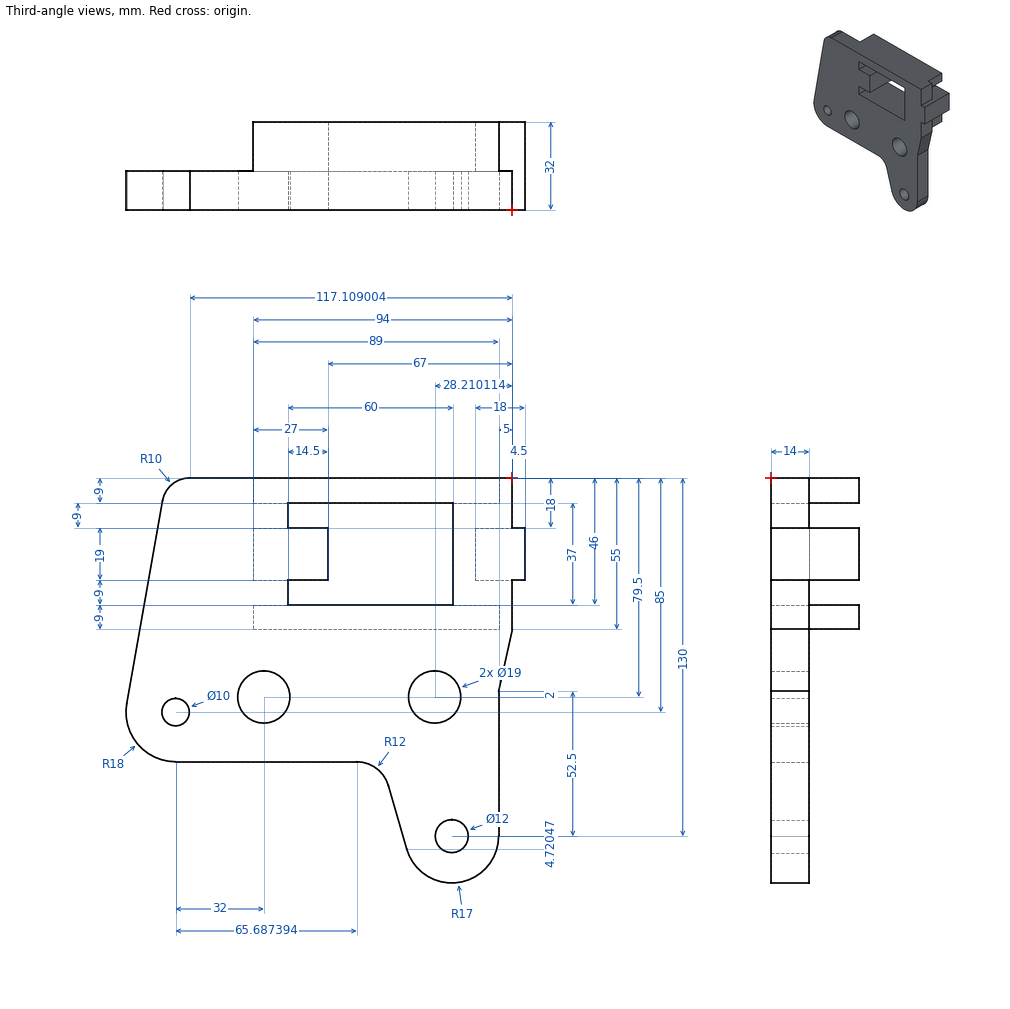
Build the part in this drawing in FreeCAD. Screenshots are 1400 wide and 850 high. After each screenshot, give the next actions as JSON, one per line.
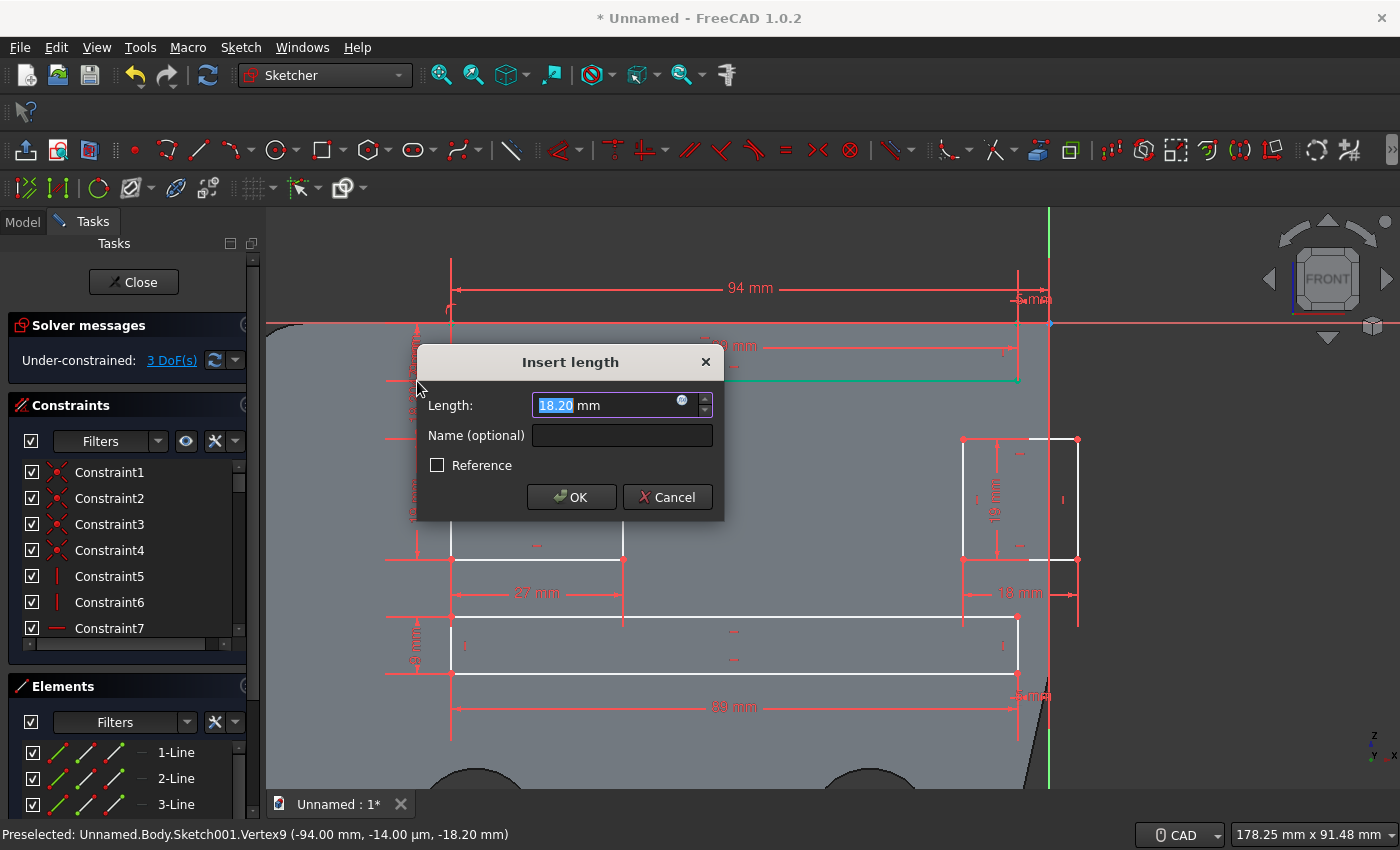
{"action": "type", "text": "18"}
{"action": "key", "text": "Return"}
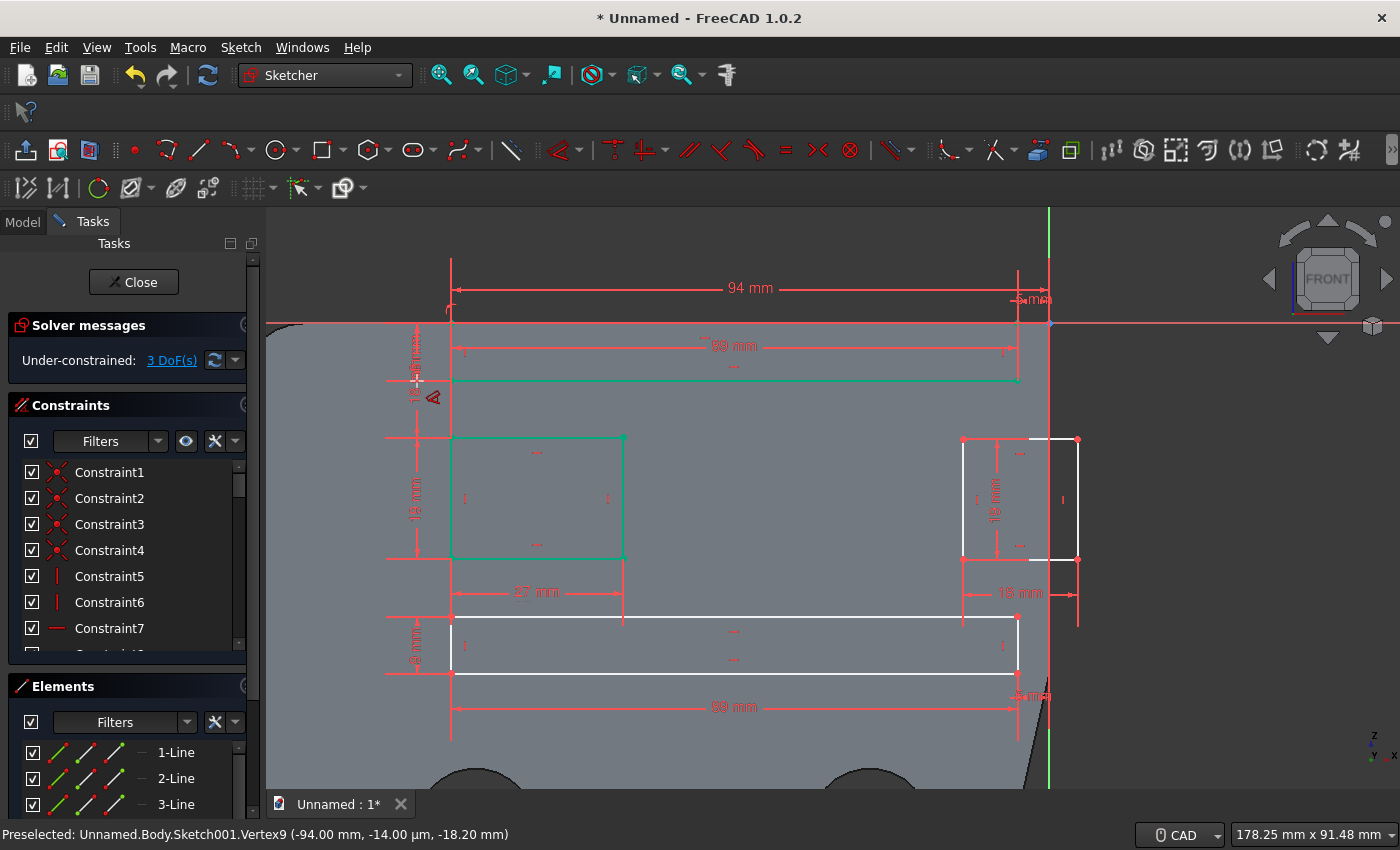
{"action": "left_click", "coordinate": [451, 617]}
{"action": "left_click", "coordinate": [417, 470]}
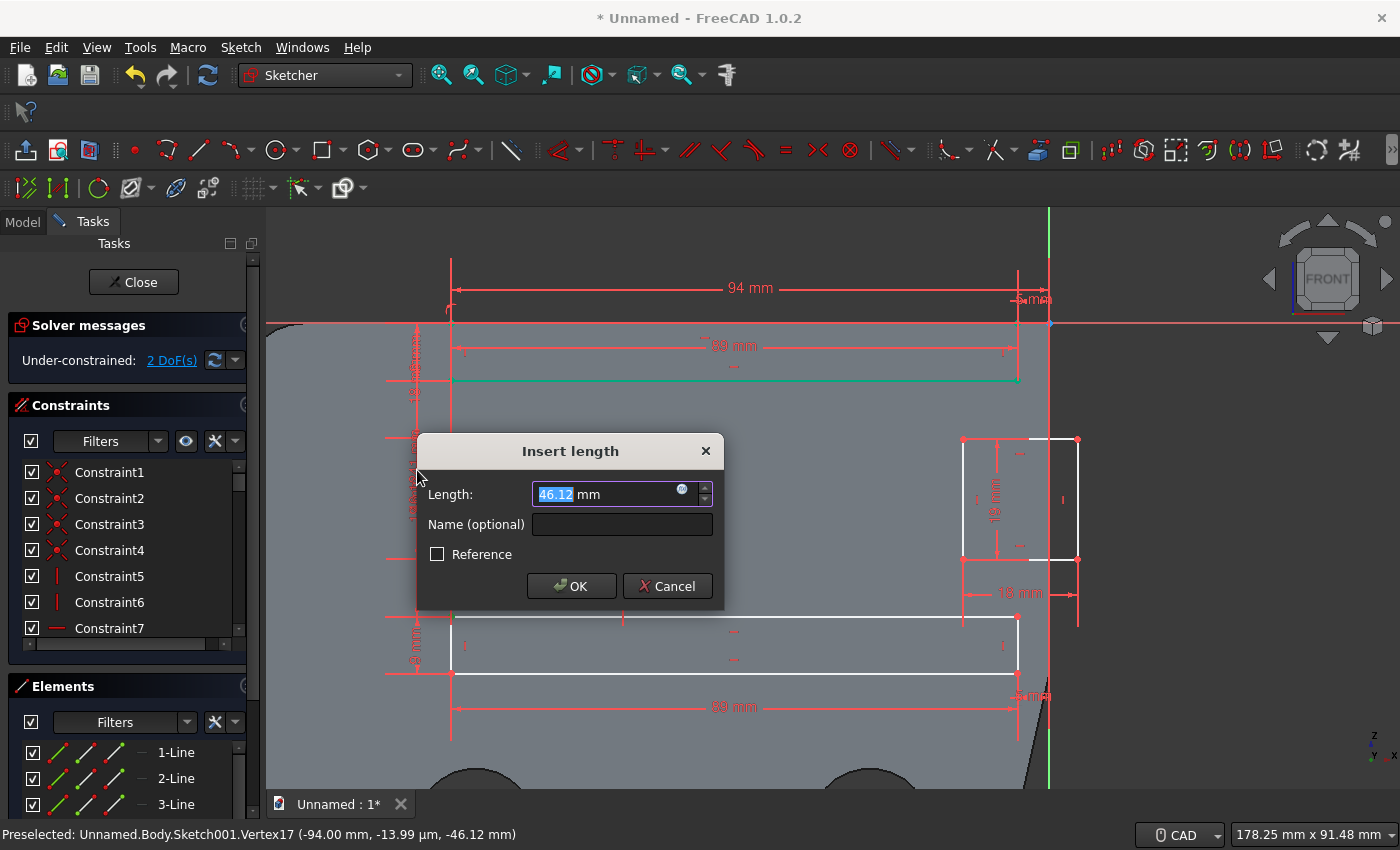
{"action": "type", "text": "46"}
{"action": "key", "text": "Return"}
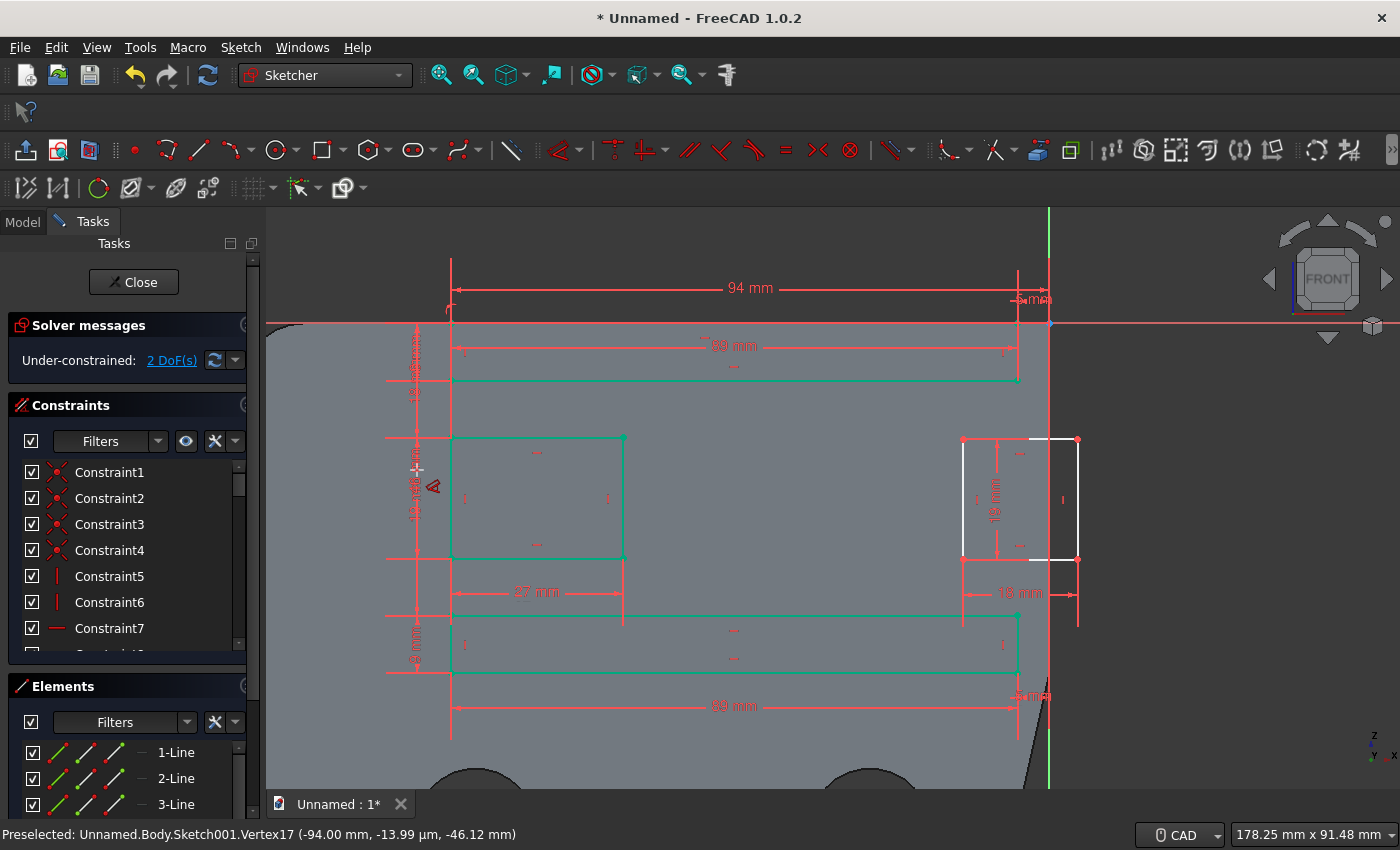
{"action": "left_click", "coordinate": [963, 439]}
{"action": "left_click", "coordinate": [1083, 381]}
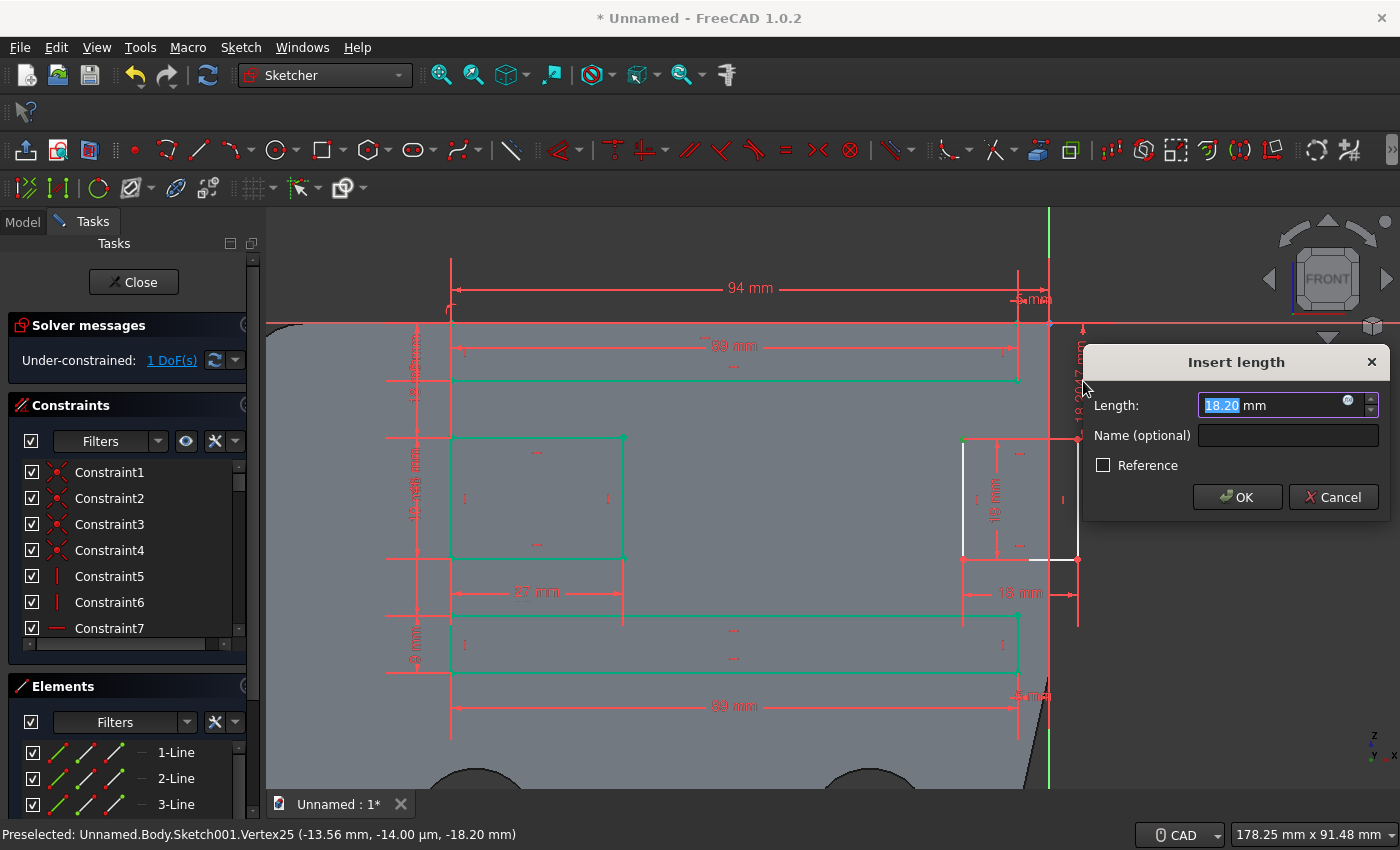
{"action": "type", "text": "18"}
{"action": "key", "text": "Return"}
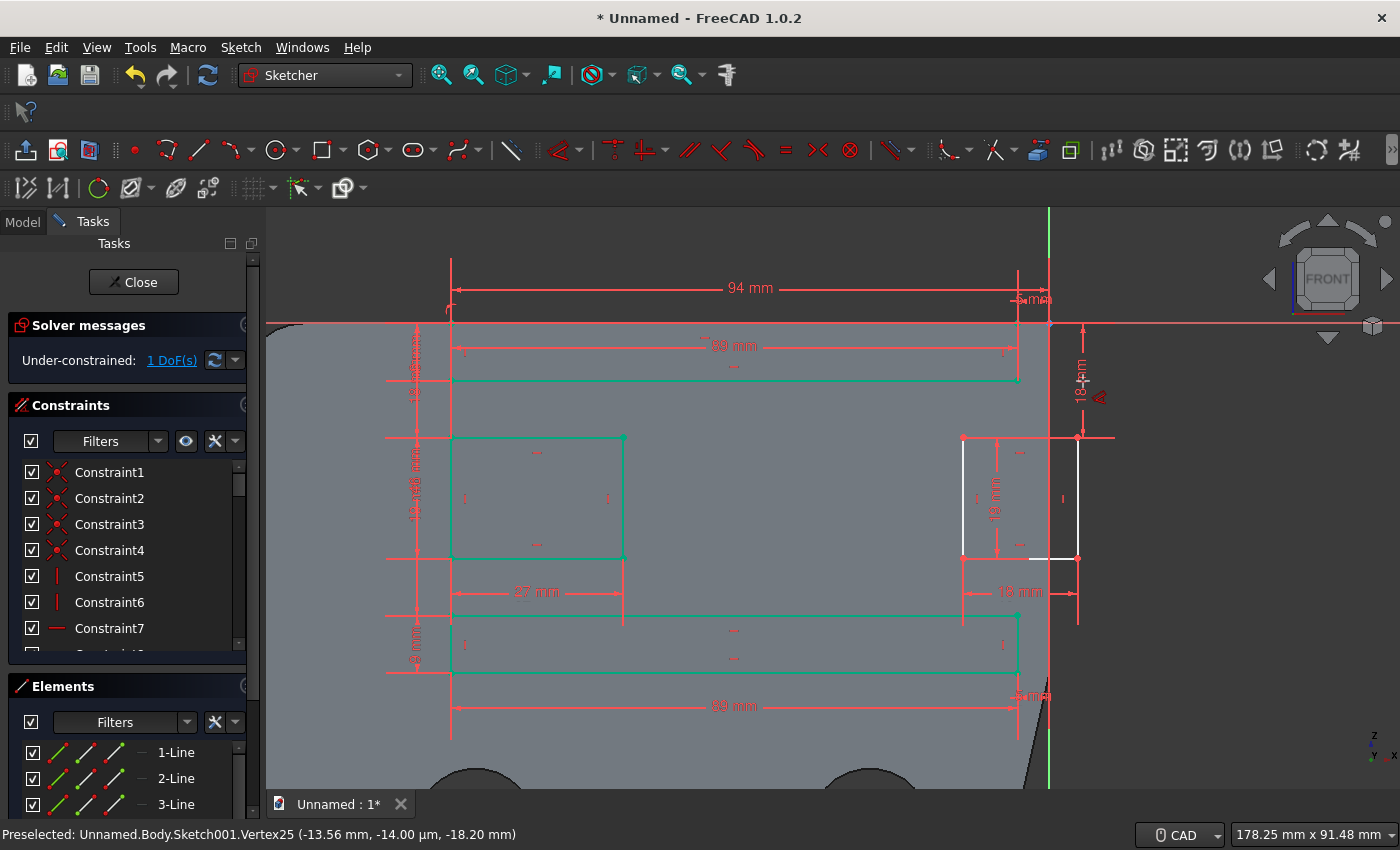
{"action": "scroll", "coordinate": [1078, 559], "scroll_direction": "up", "scroll_amount": 2}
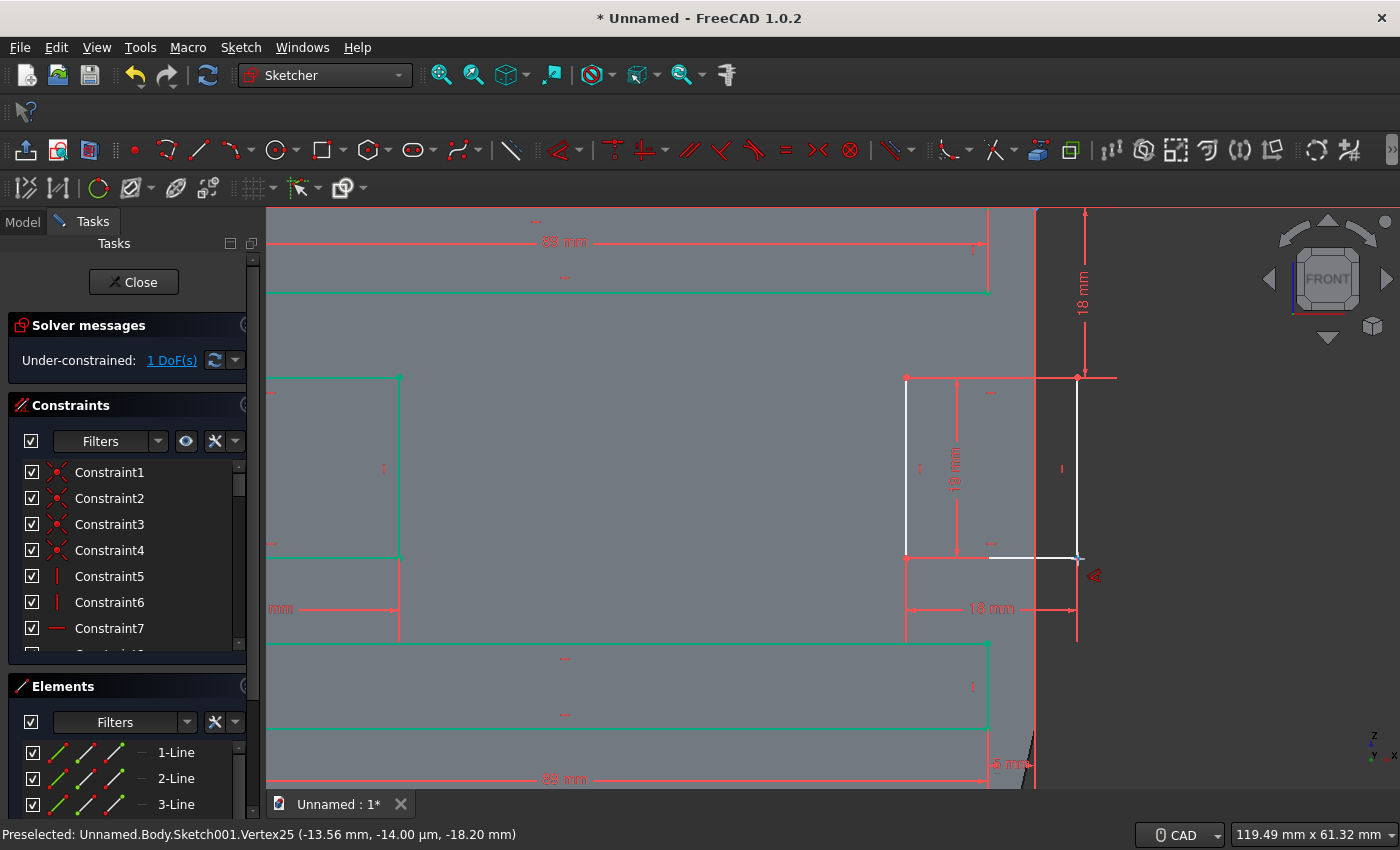
{"action": "left_click", "coordinate": [1077, 558]}
{"action": "left_click", "coordinate": [1066, 592]}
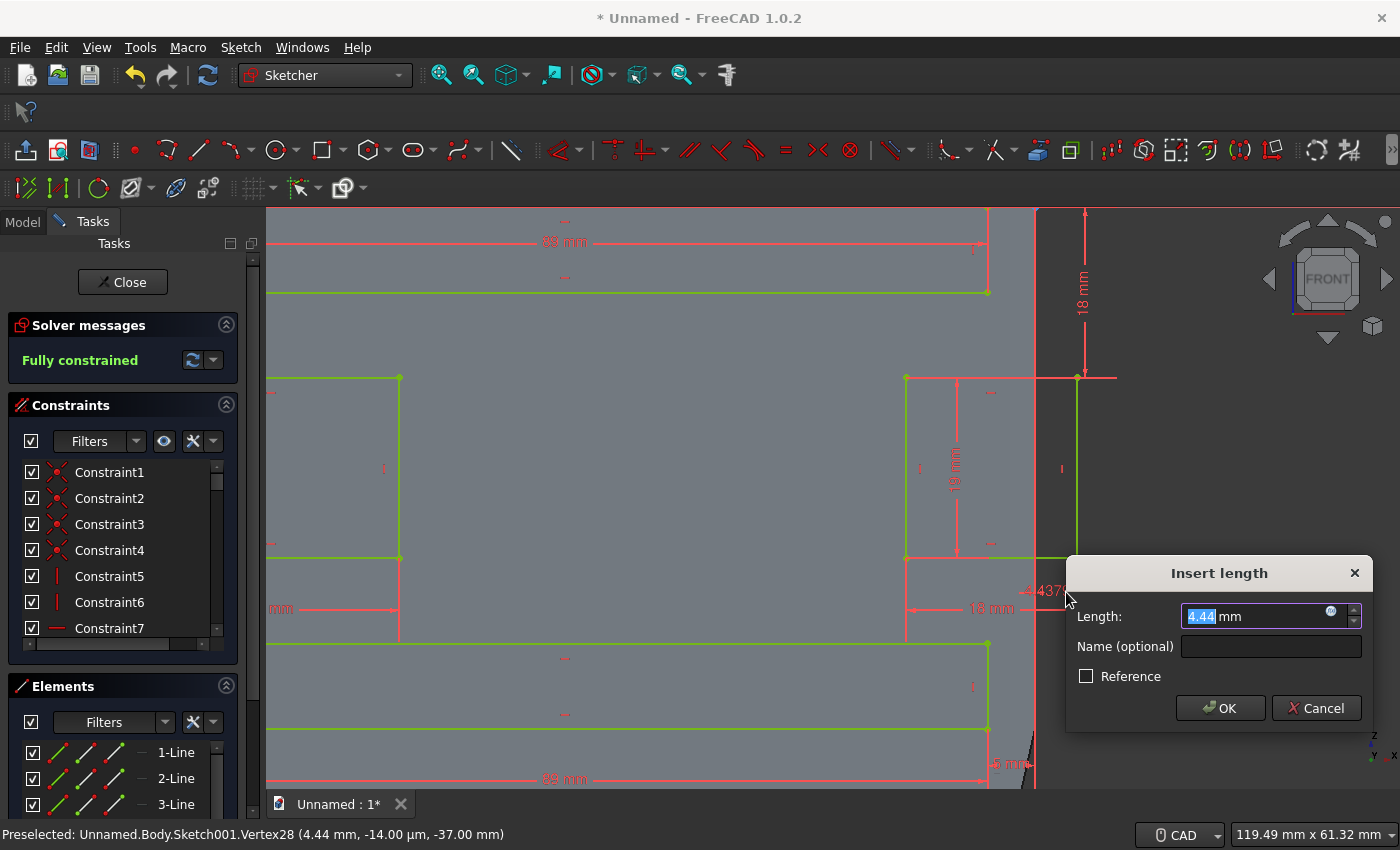
{"action": "type", "text": "4.5"}
{"action": "key", "text": "Return"}
{"action": "key", "text": "Escape"}